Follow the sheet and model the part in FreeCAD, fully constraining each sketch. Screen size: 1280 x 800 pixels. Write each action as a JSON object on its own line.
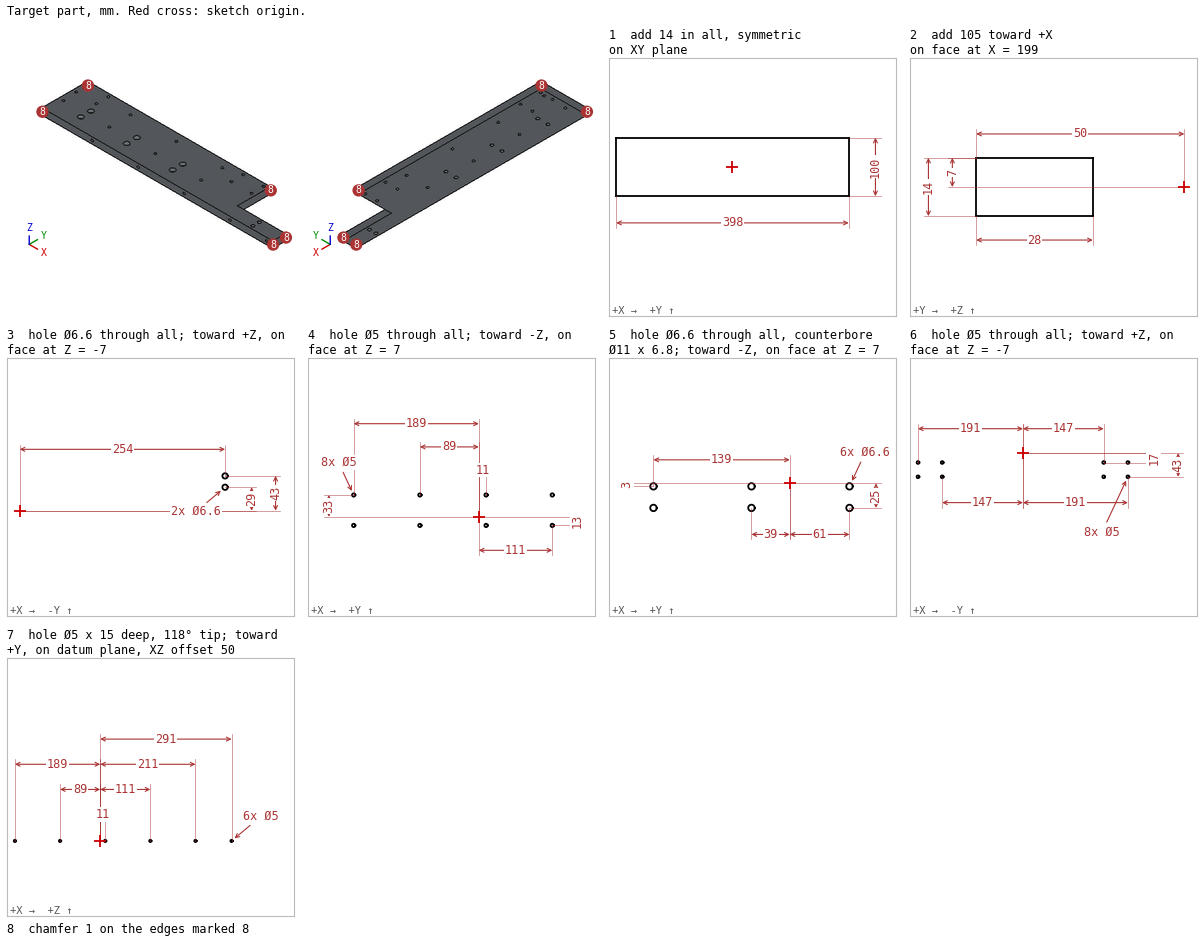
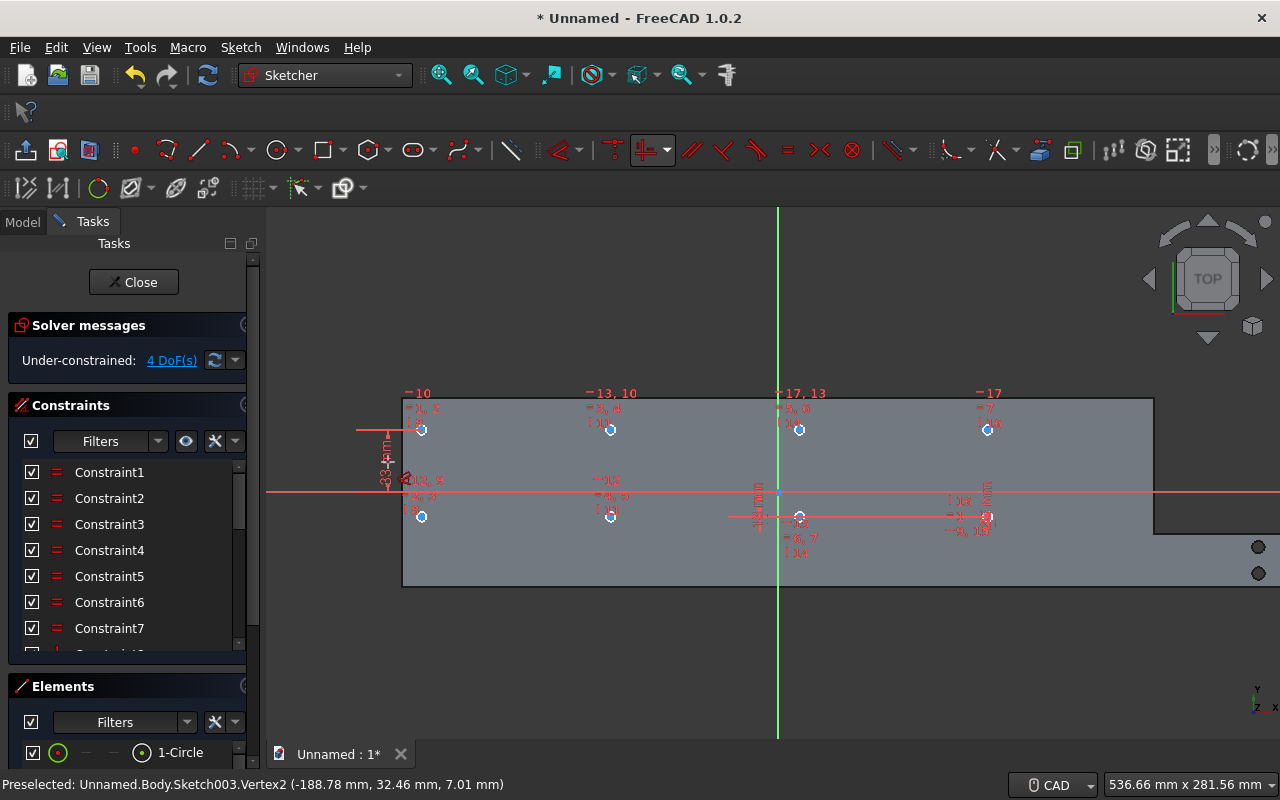
{"action": "left_click", "coordinate": [611, 430]}
{"action": "left_click", "coordinate": [695, 396]}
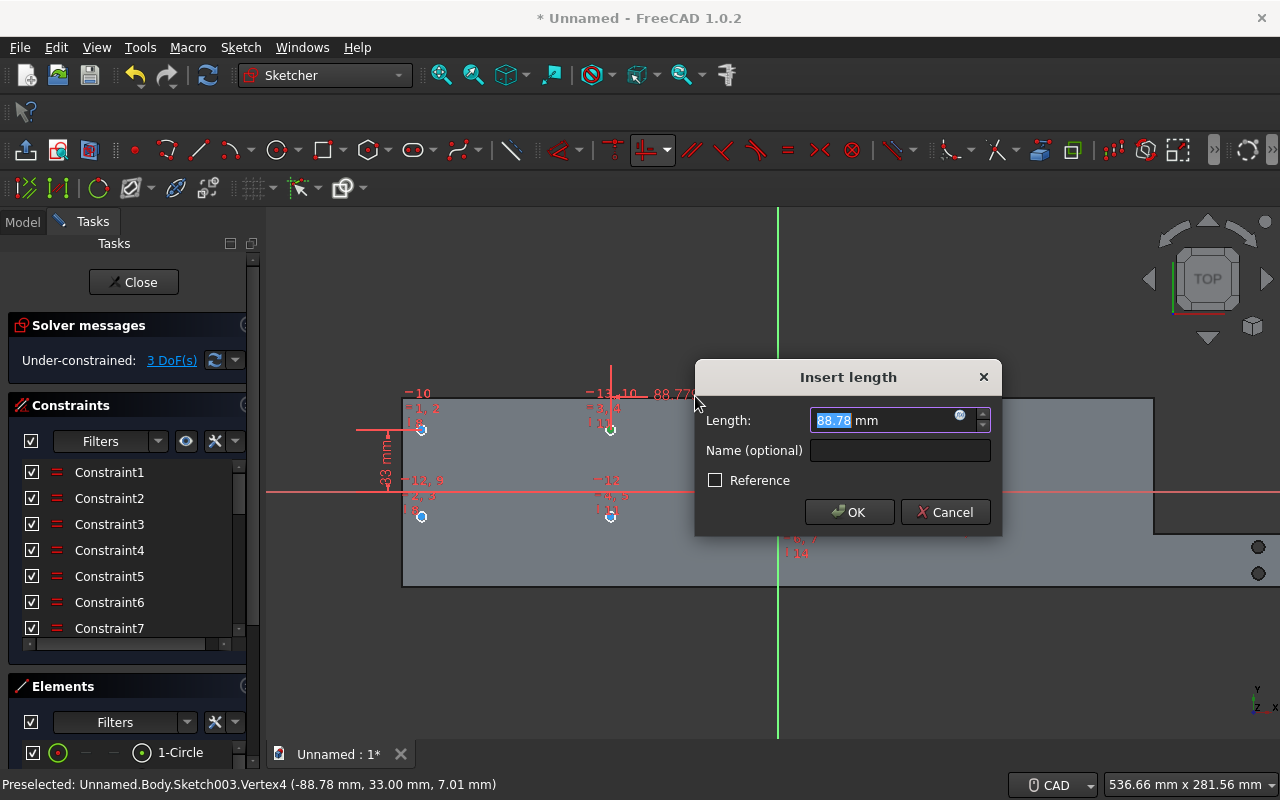
{"action": "type", "text": "89"}
{"action": "key", "text": "Return"}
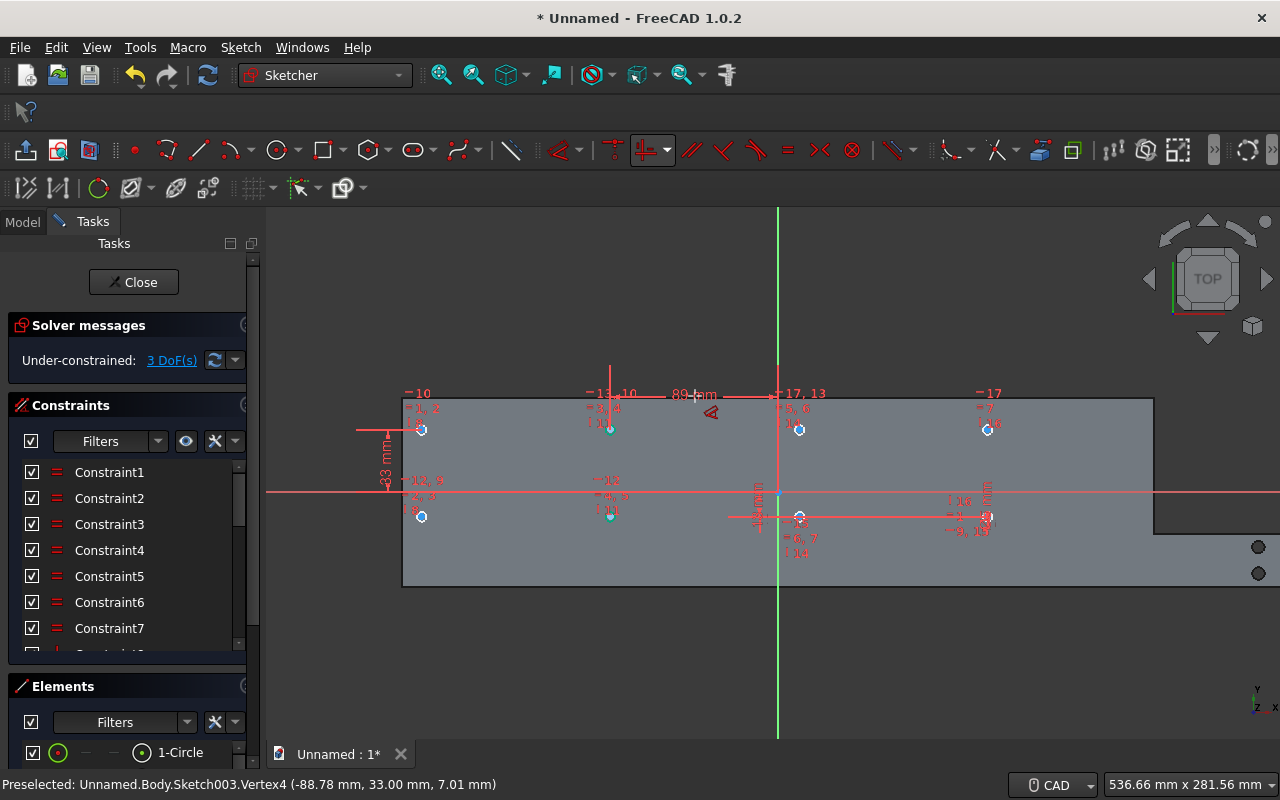
{"action": "scroll", "coordinate": [800, 430], "scroll_direction": "up", "scroll_amount": 4}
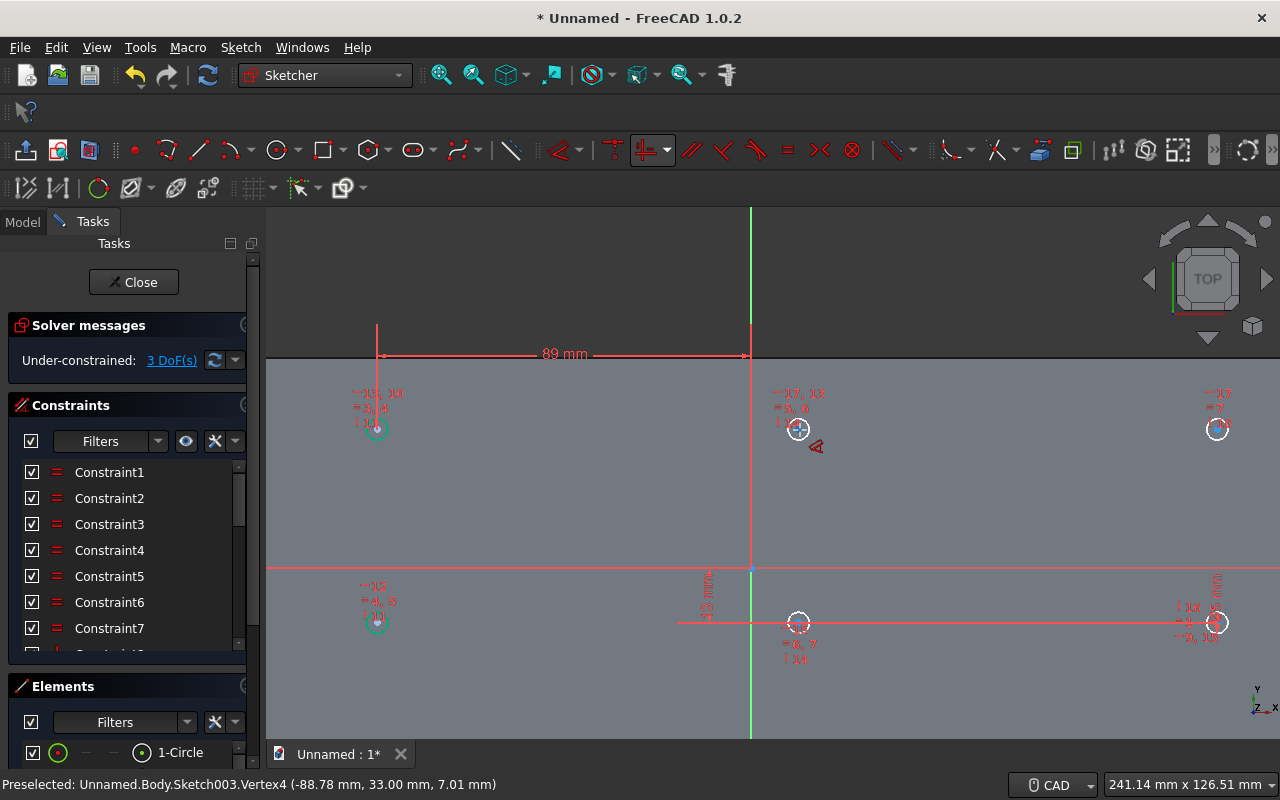
{"action": "left_click", "coordinate": [799, 429]}
{"action": "left_click", "coordinate": [775, 395]}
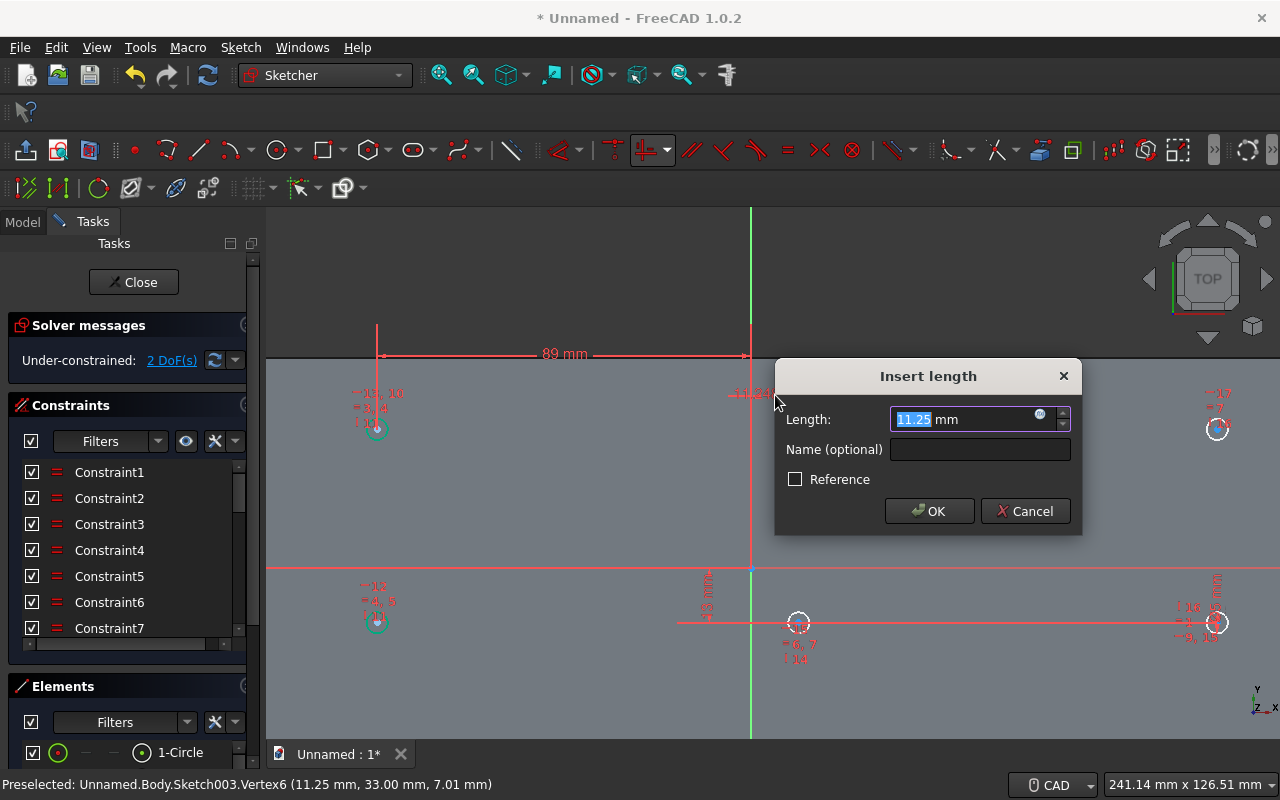
{"action": "type", "text": "11"}
{"action": "key", "text": "Return"}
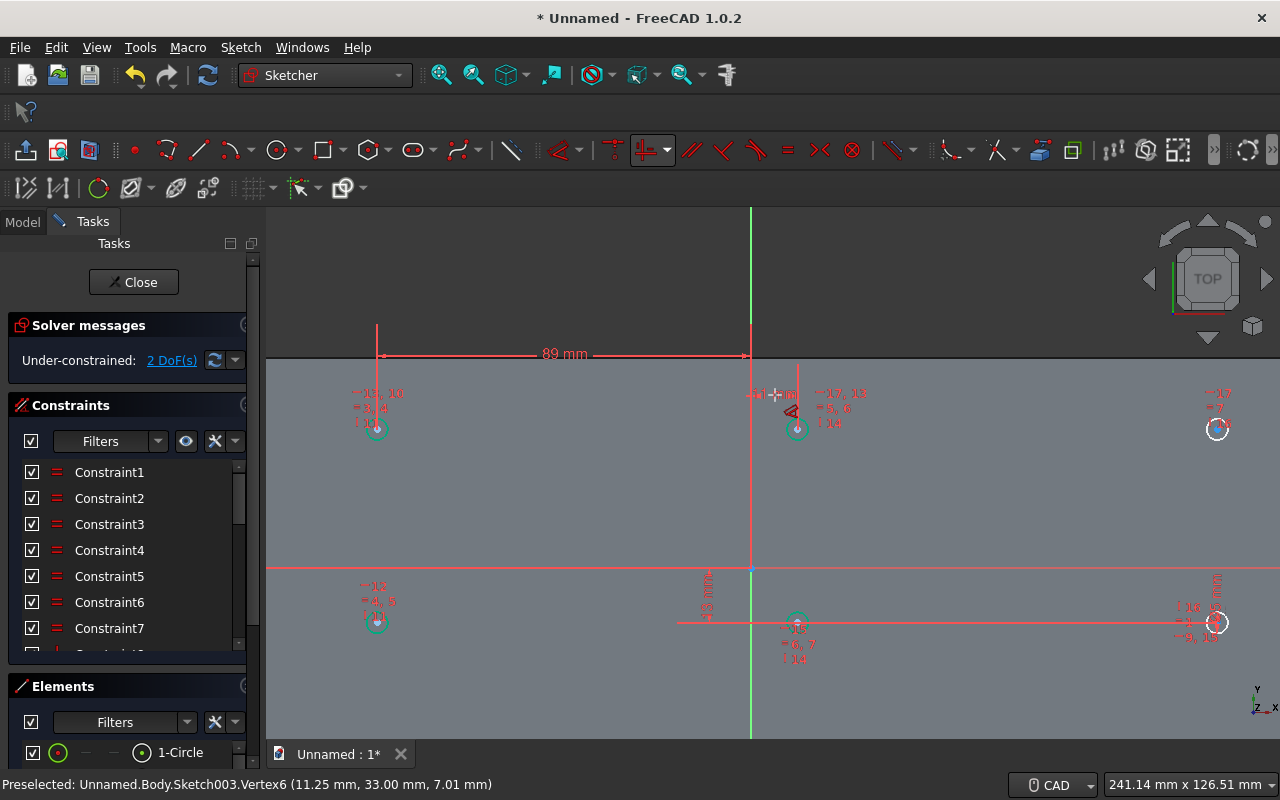
{"action": "scroll", "coordinate": [800, 430], "scroll_direction": "down", "scroll_amount": 4}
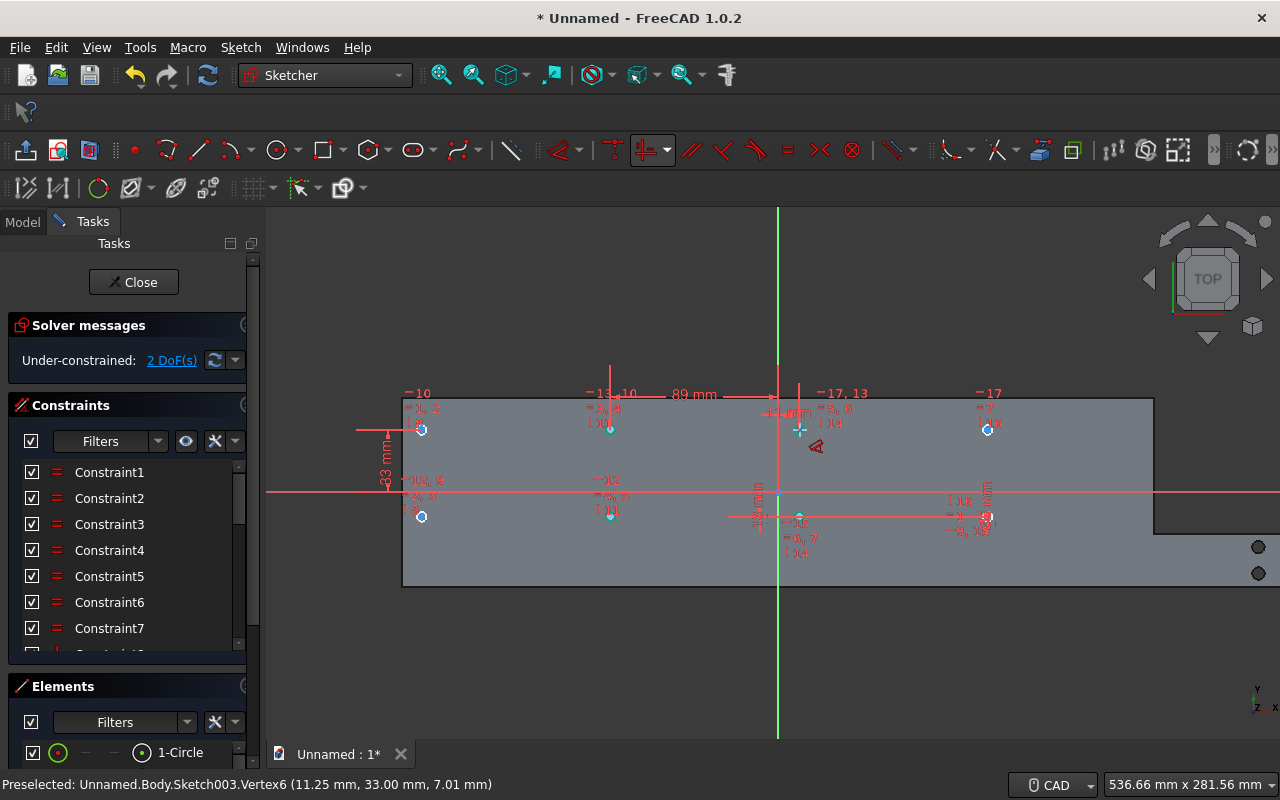
{"action": "left_click", "coordinate": [988, 517]}
{"action": "left_click", "coordinate": [883, 551]}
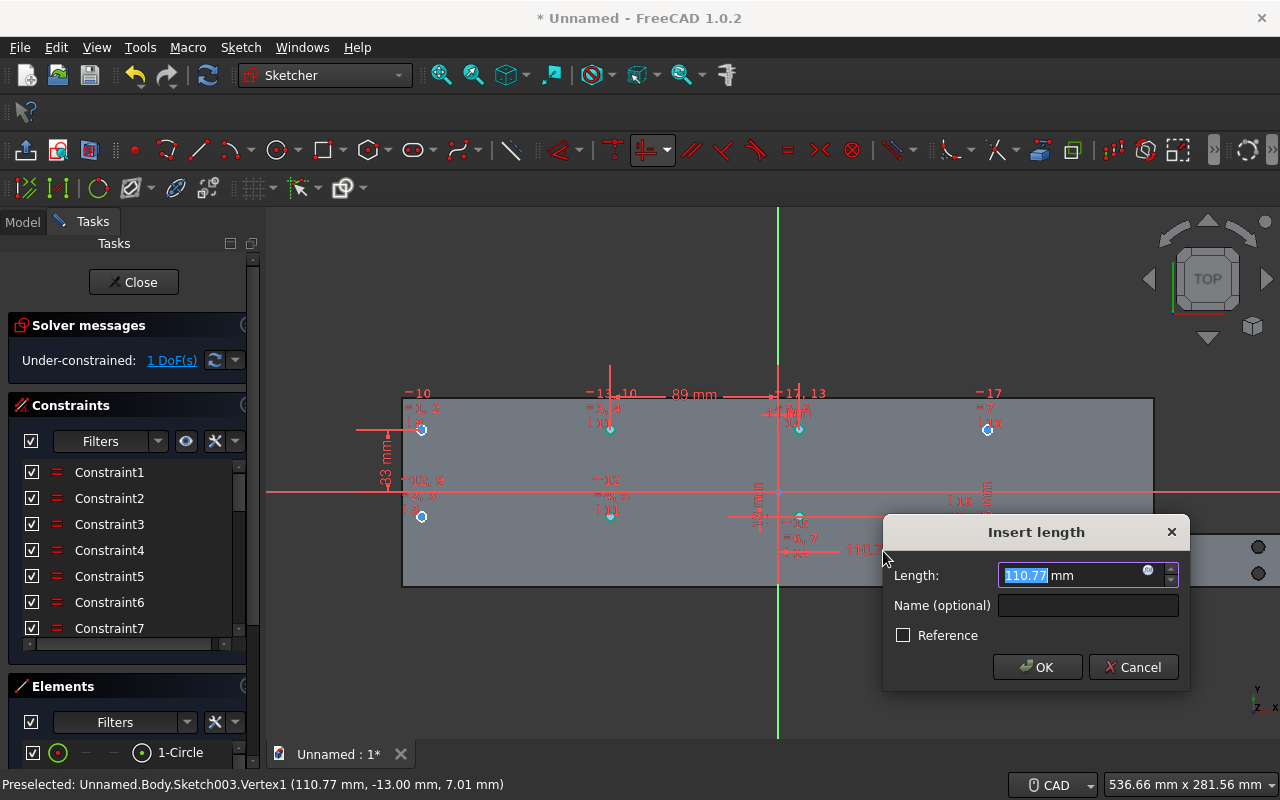
{"action": "type", "text": "111"}
{"action": "key", "text": "Return"}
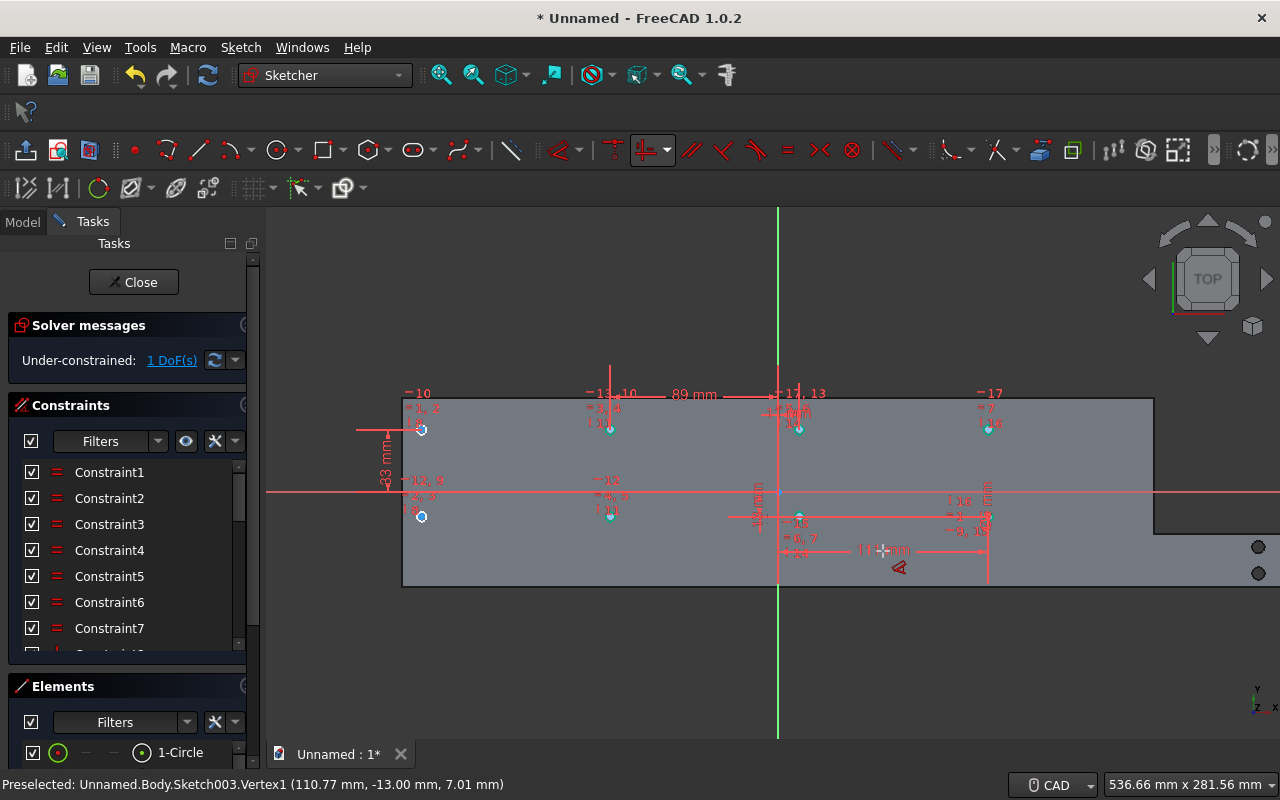
{"action": "left_click", "coordinate": [422, 430]}
{"action": "left_click", "coordinate": [600, 396]}